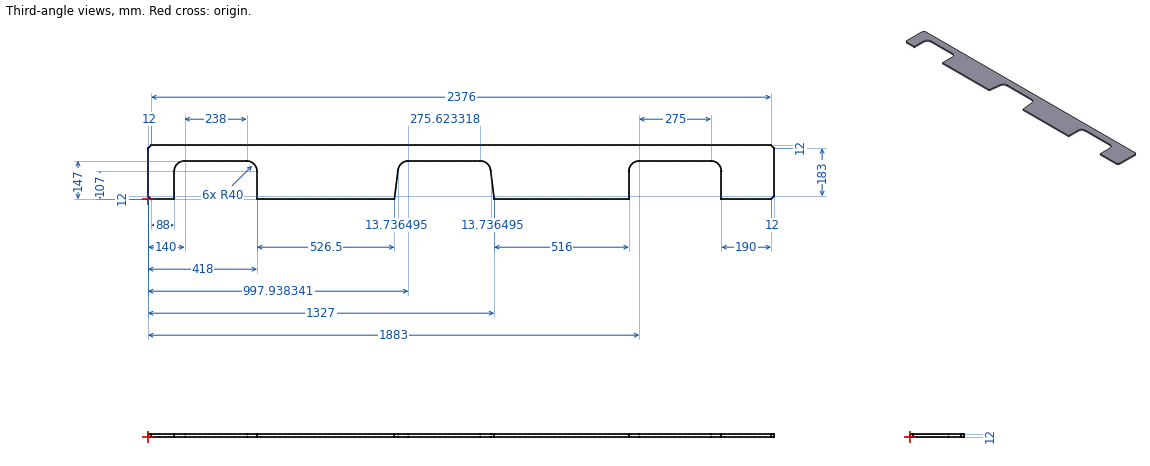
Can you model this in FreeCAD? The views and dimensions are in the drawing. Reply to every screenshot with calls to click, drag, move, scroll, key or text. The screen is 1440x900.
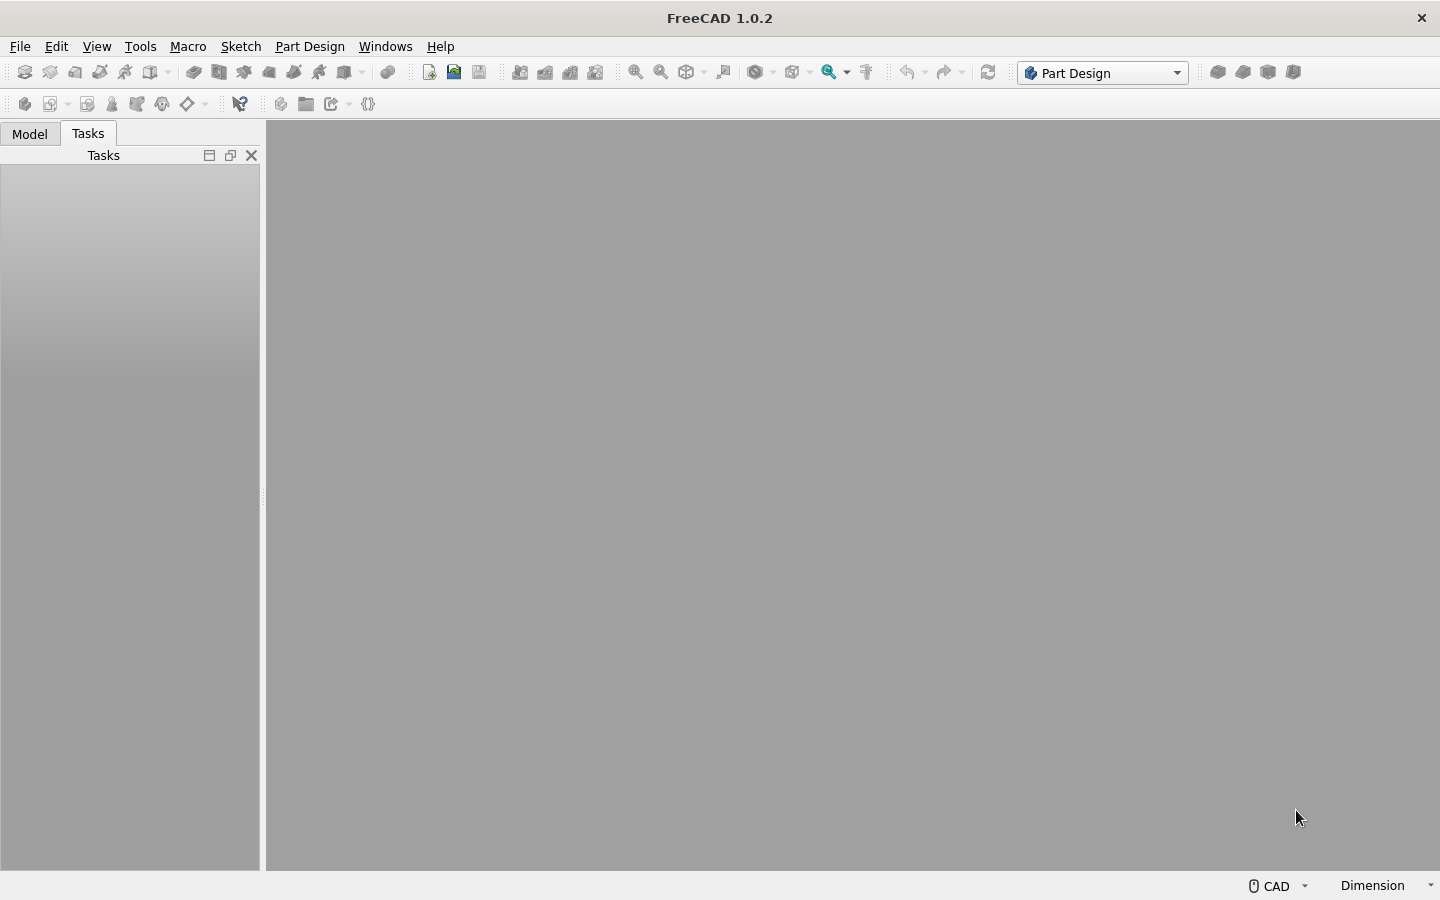
click(429, 72)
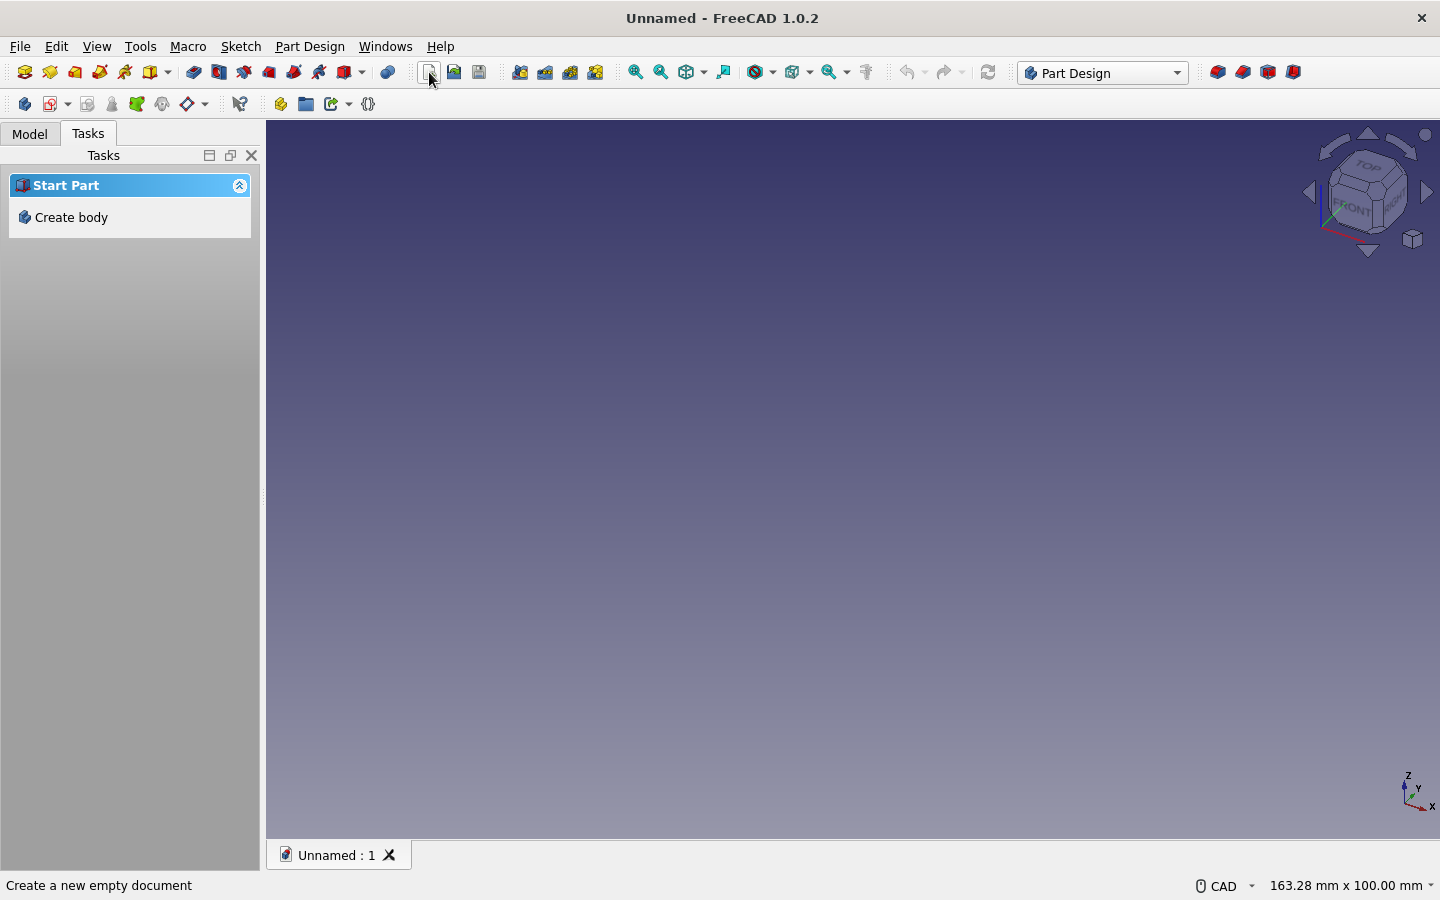
click(50, 104)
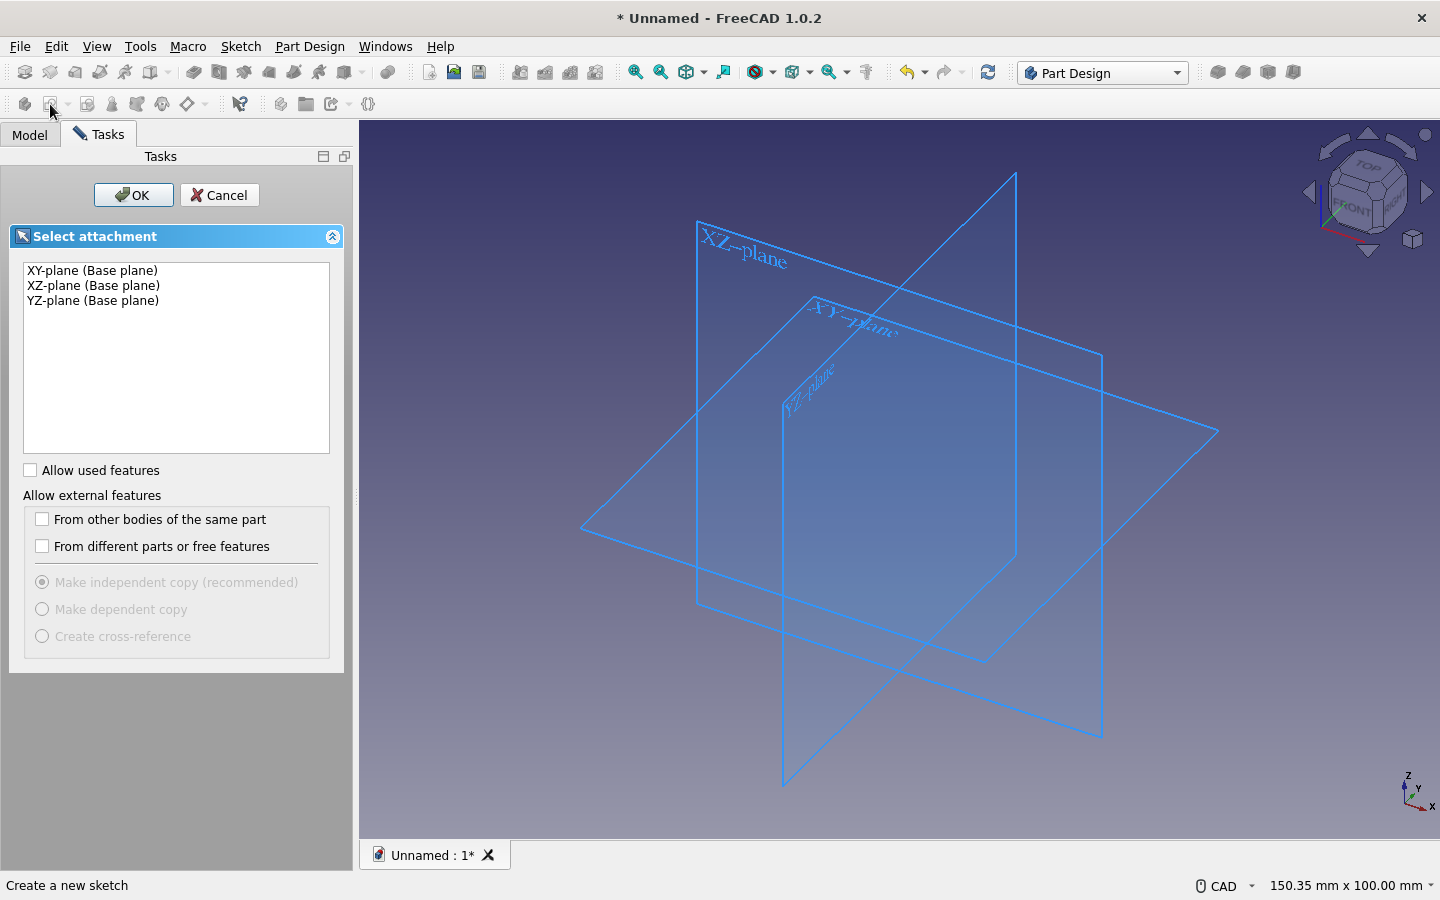
click(84, 270)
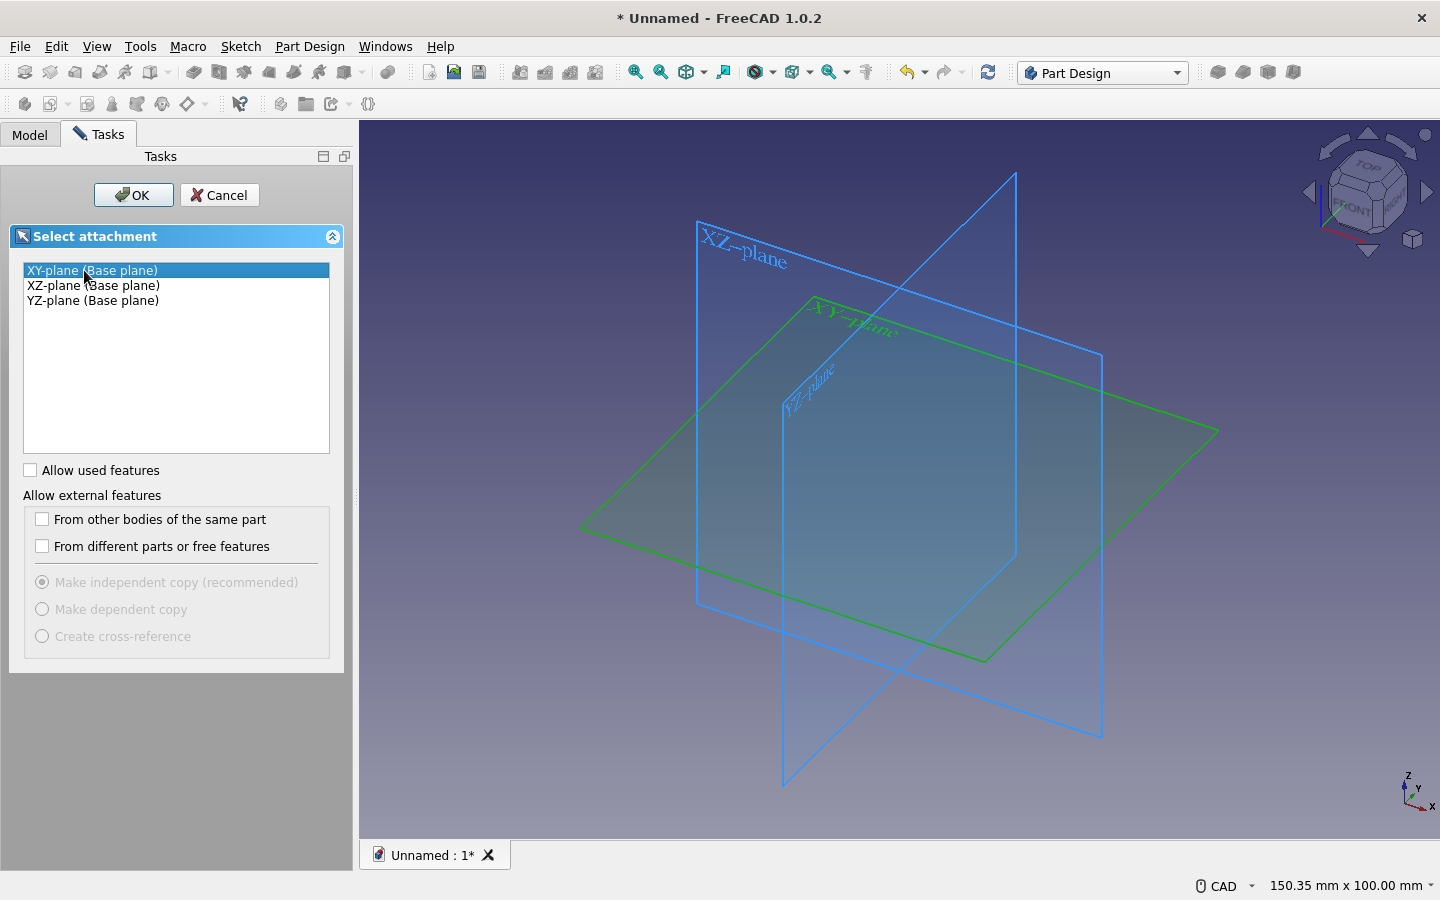
click(134, 195)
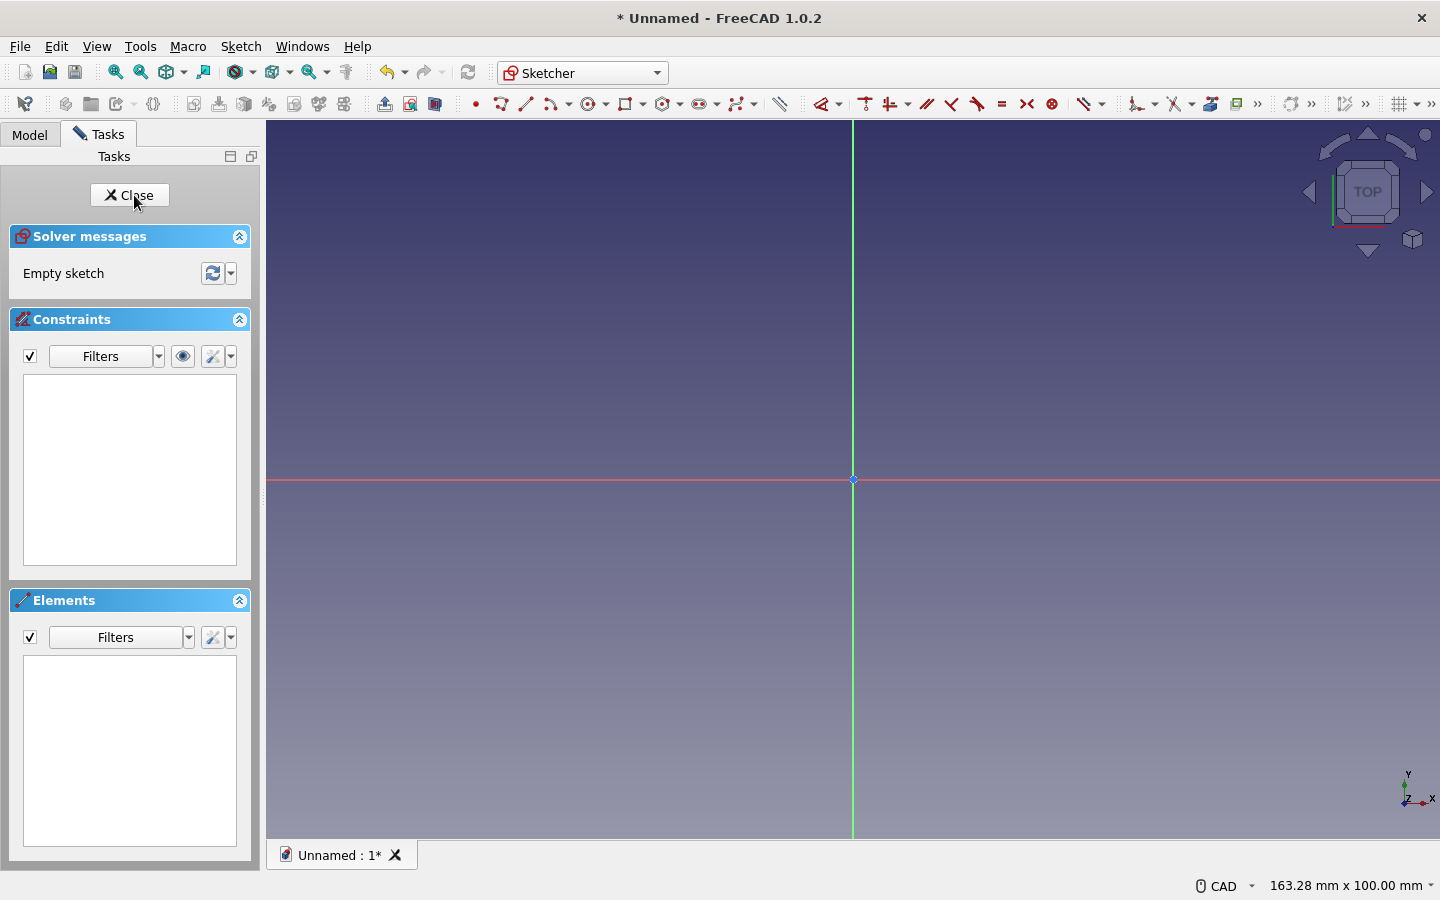
scroll(329, 518, down, 15)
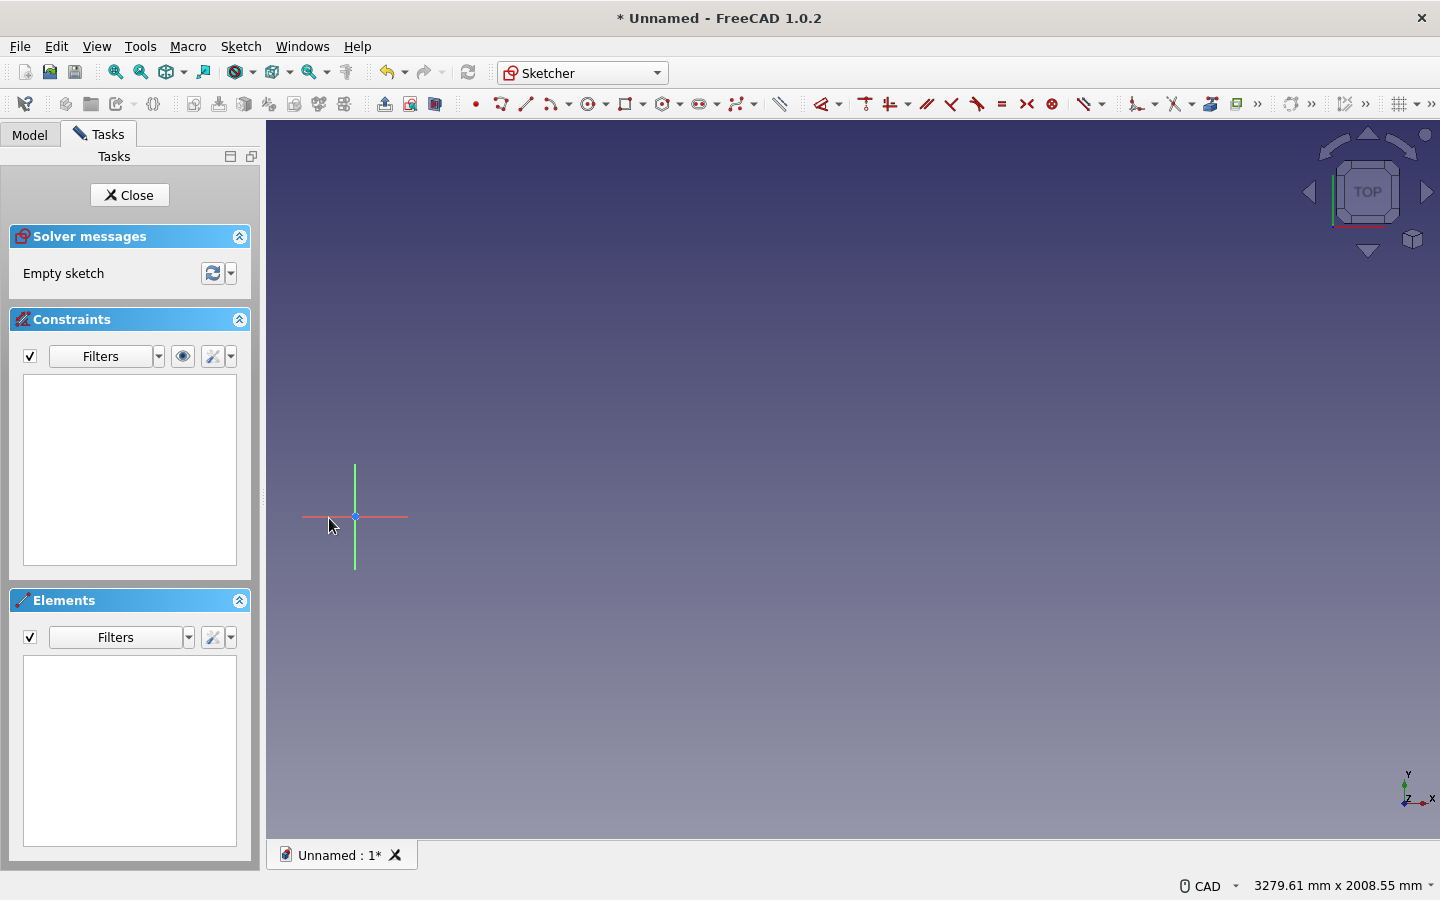
click(526, 104)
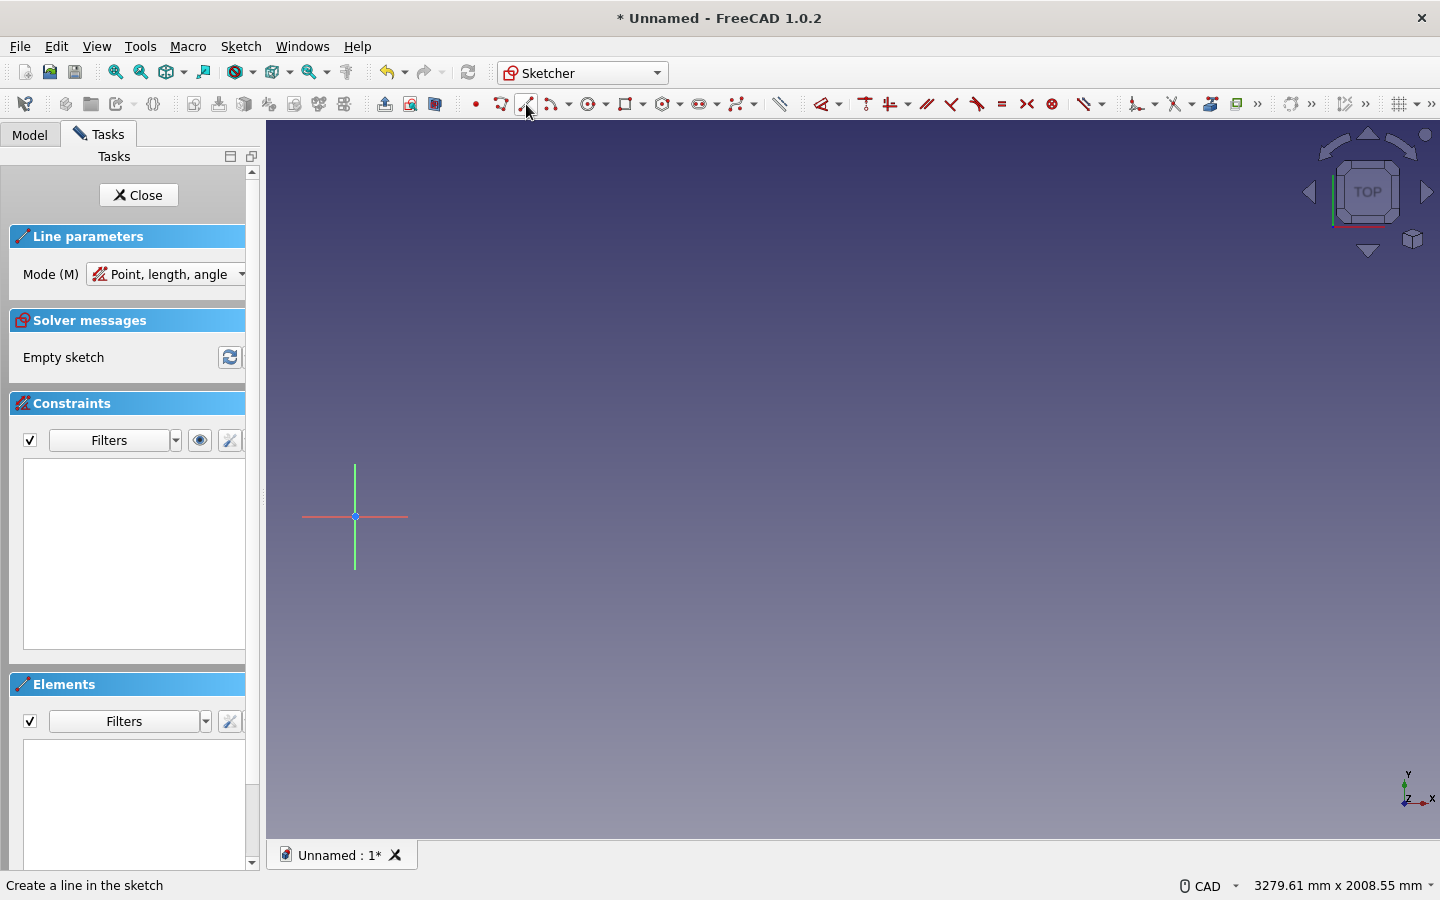
click(405, 464)
click(490, 464)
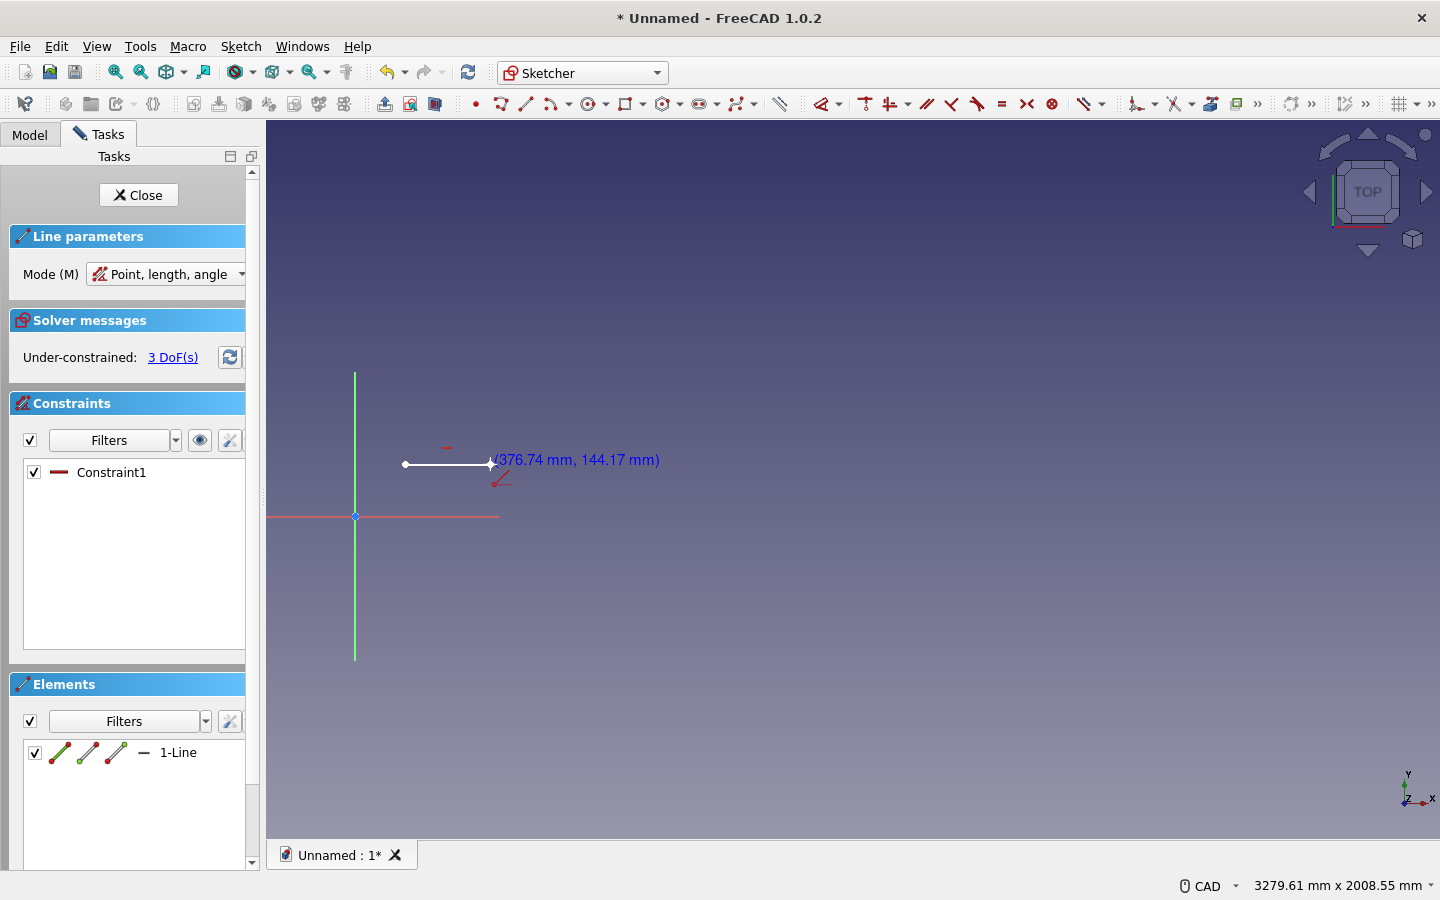
click(501, 104)